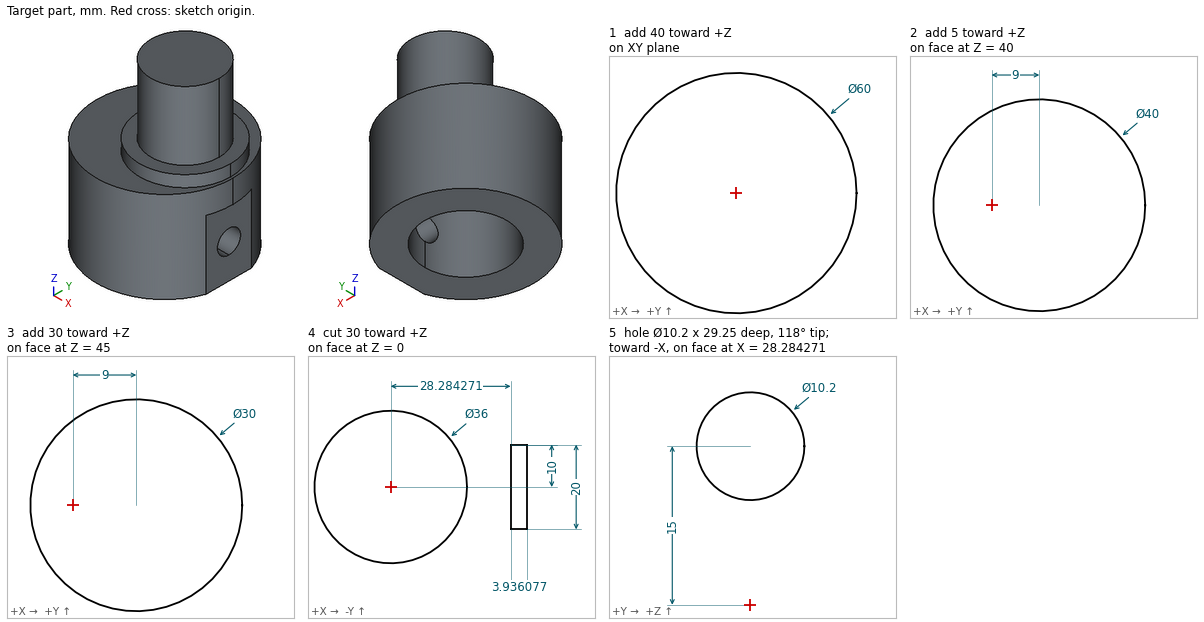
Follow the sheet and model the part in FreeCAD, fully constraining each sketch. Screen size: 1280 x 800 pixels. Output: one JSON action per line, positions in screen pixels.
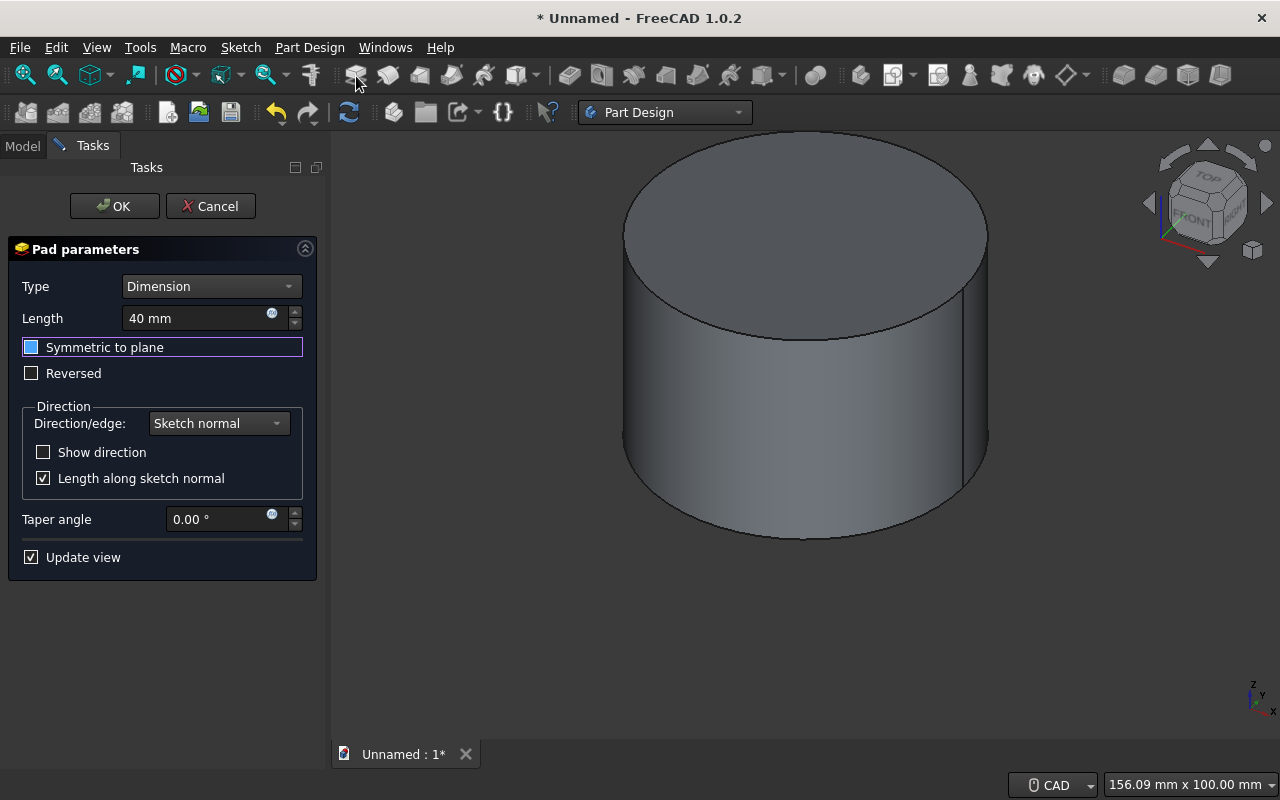
{"action": "left_click", "coordinate": [115, 206]}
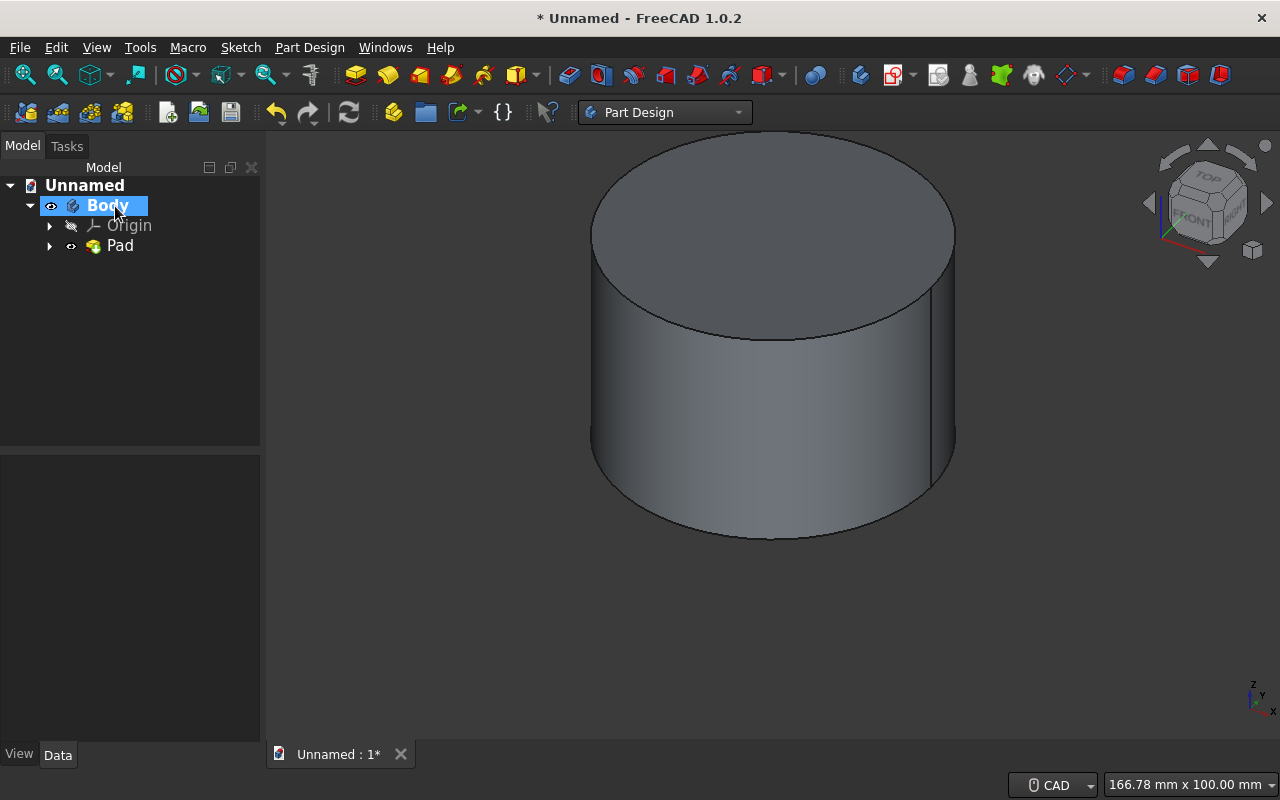
{"action": "key", "text": "v f"}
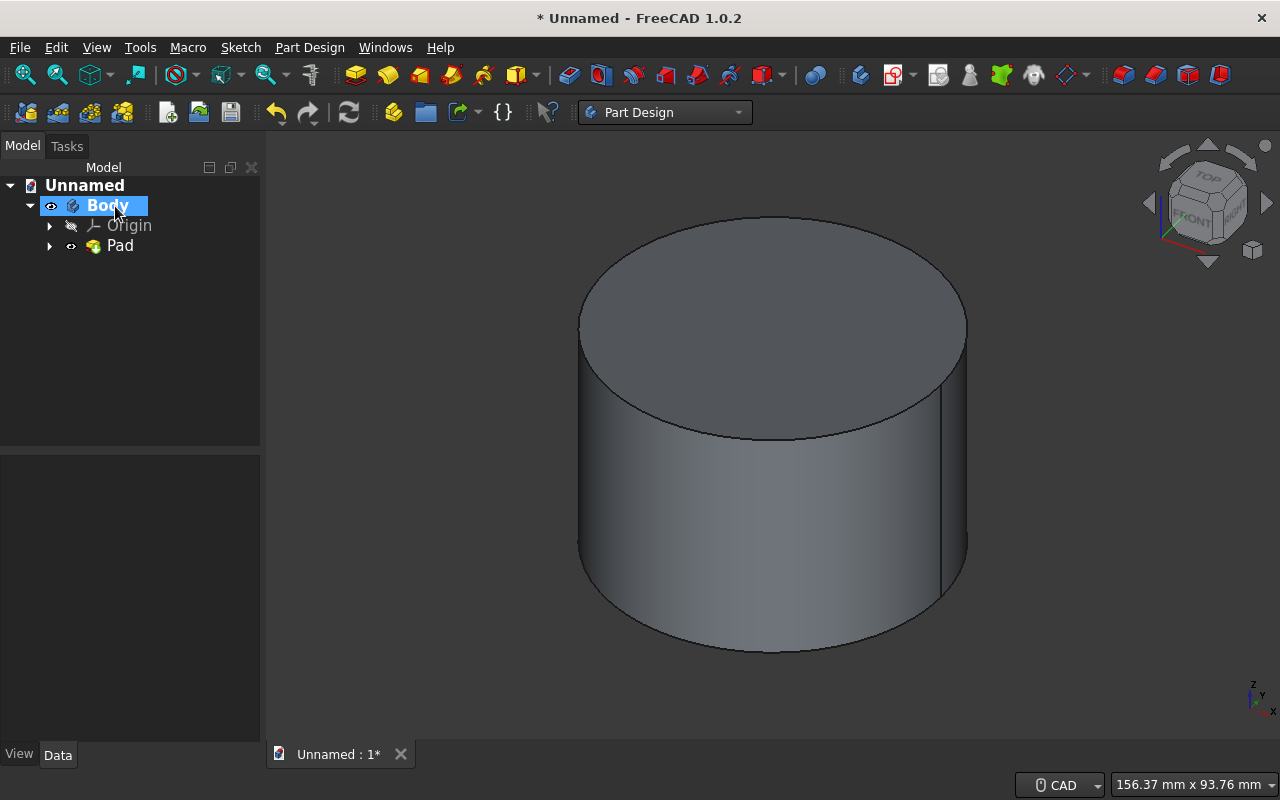
{"action": "left_click", "coordinate": [773, 328]}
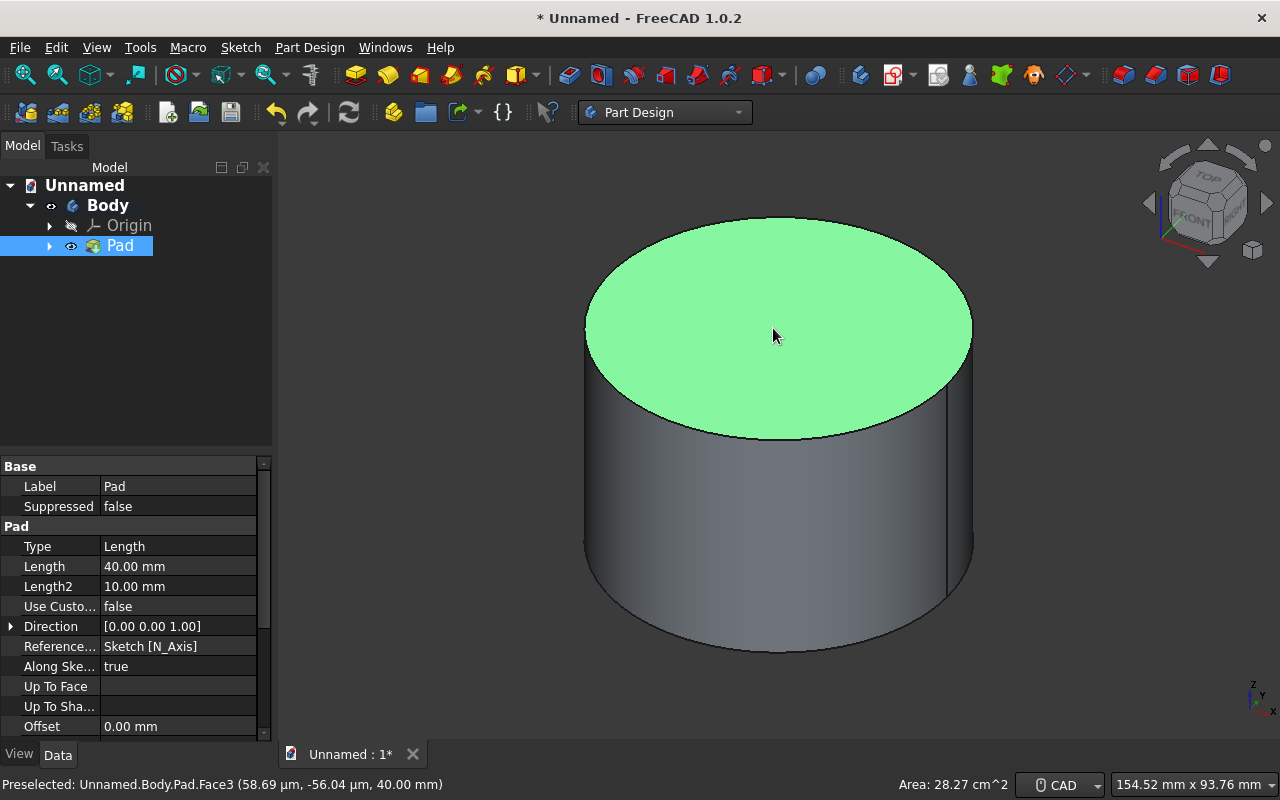
{"action": "left_click", "coordinate": [894, 76]}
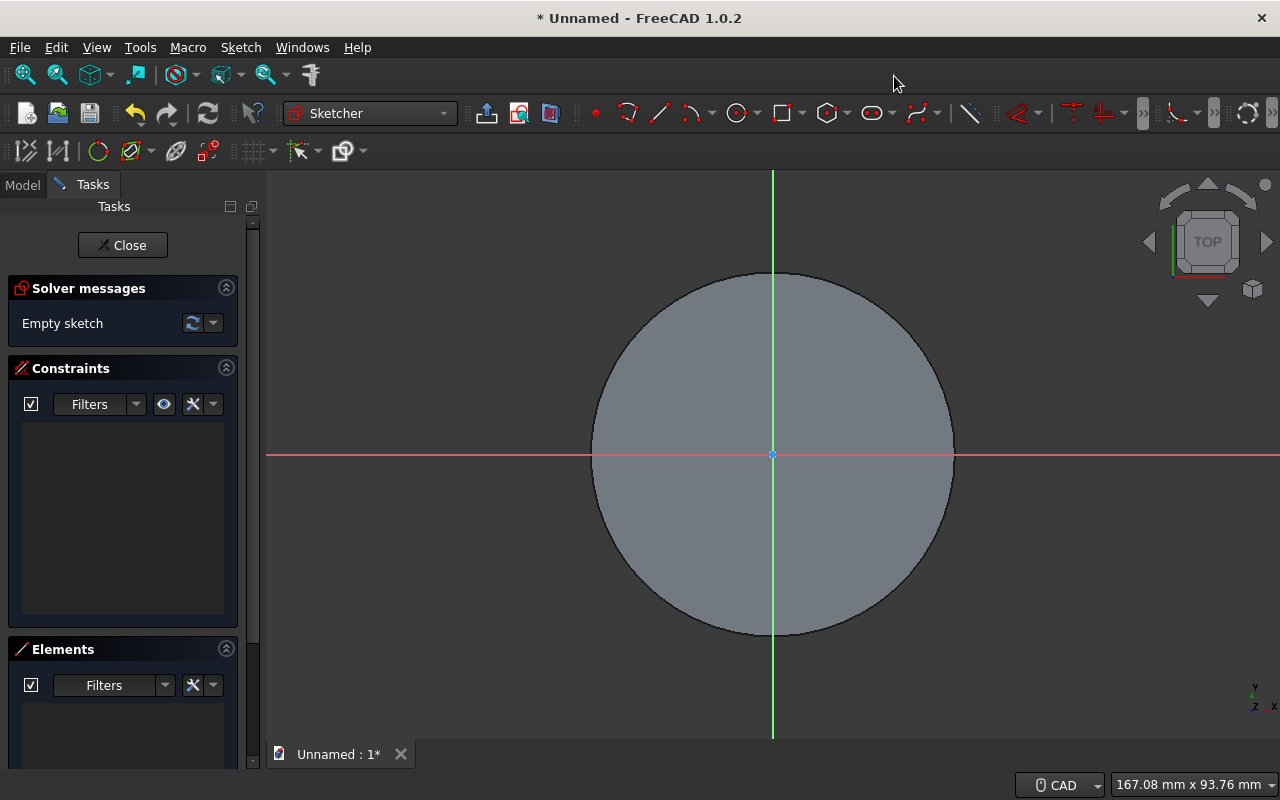
{"action": "scroll", "coordinate": [1077, 455], "scroll_direction": "up", "scroll_amount": 2}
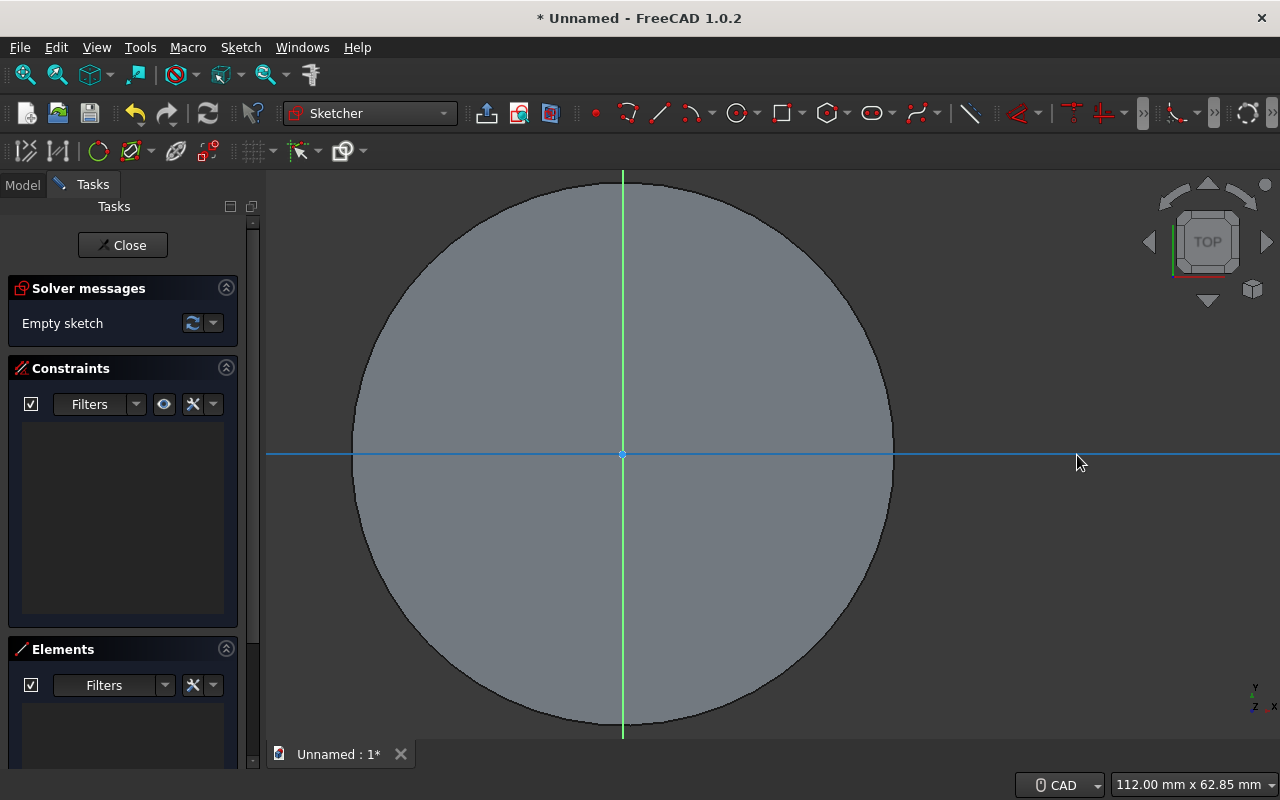
{"action": "left_click", "coordinate": [738, 114]}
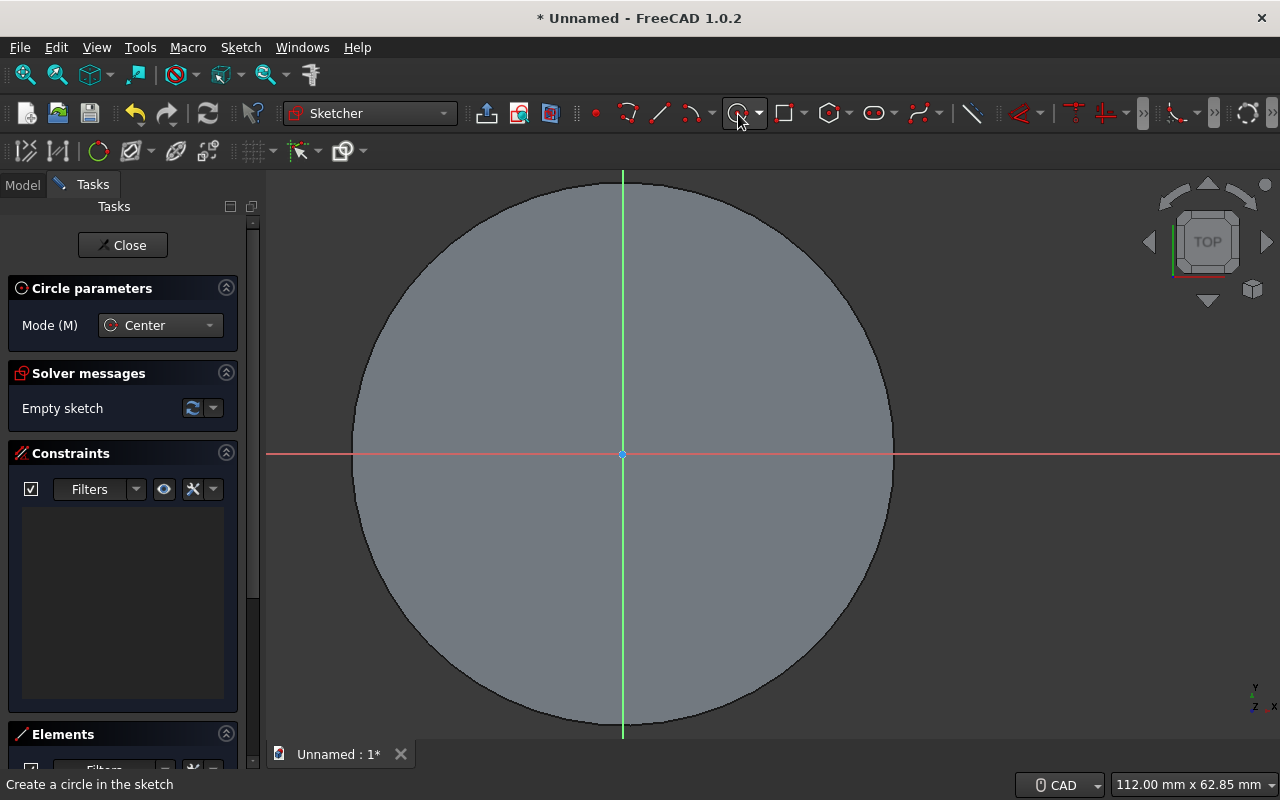
{"action": "left_click", "coordinate": [704, 454]}
{"action": "mouse_move", "coordinate": [832, 326]}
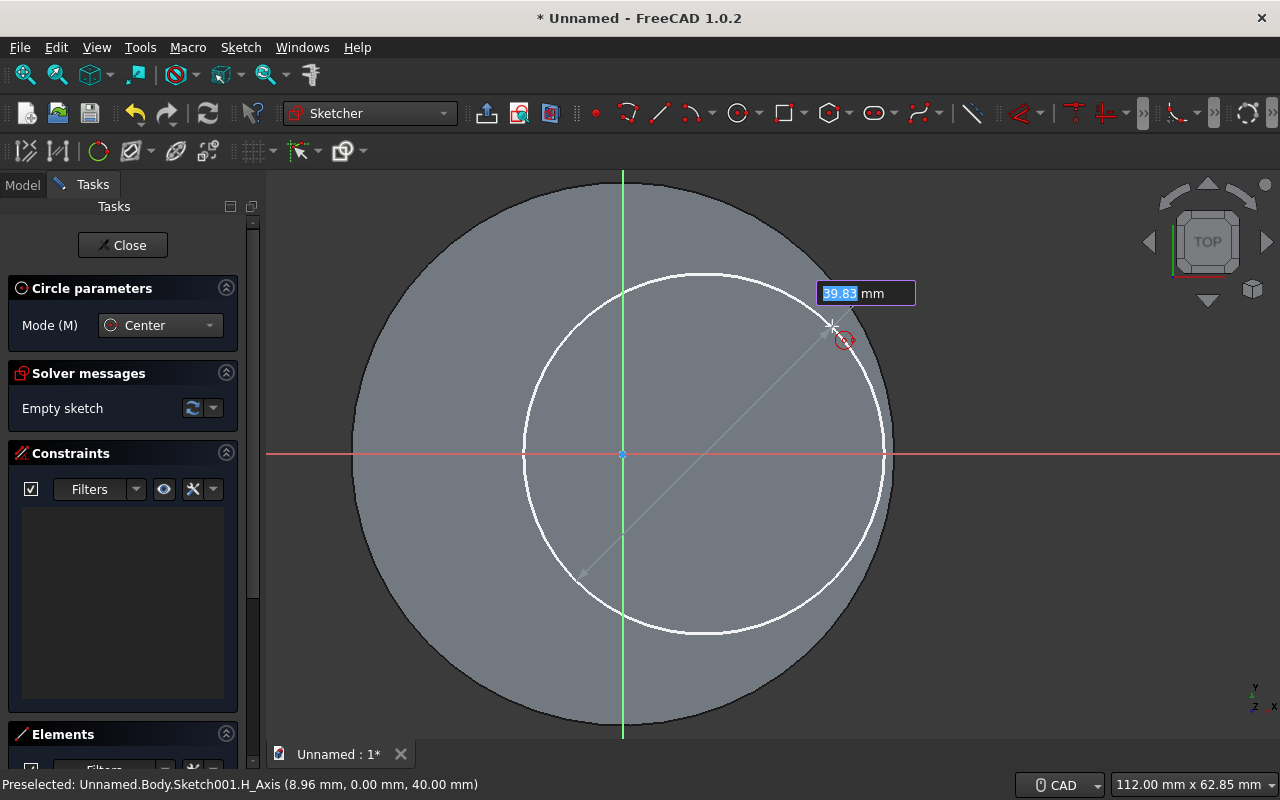
{"action": "type", "text": "40"}
{"action": "key", "text": "Return"}
{"action": "key", "text": "Escape"}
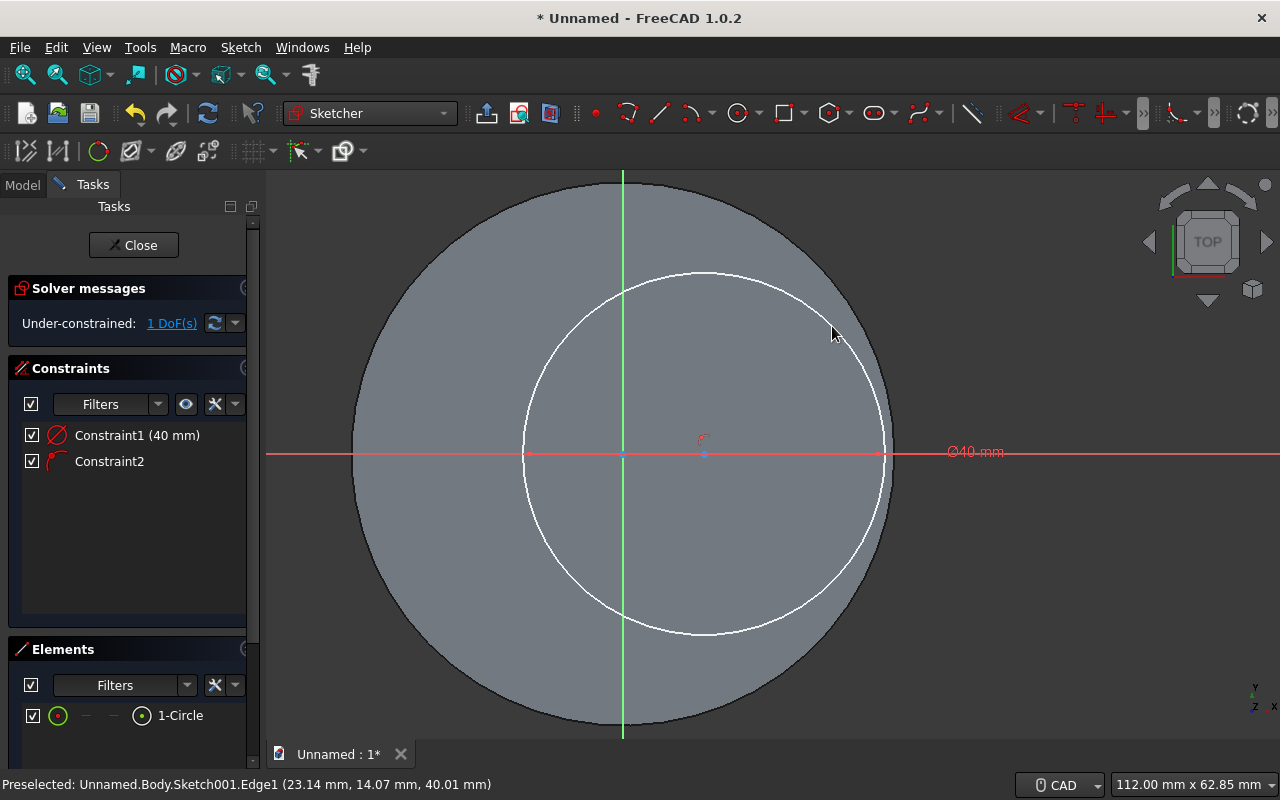
{"action": "key", "text": "d"}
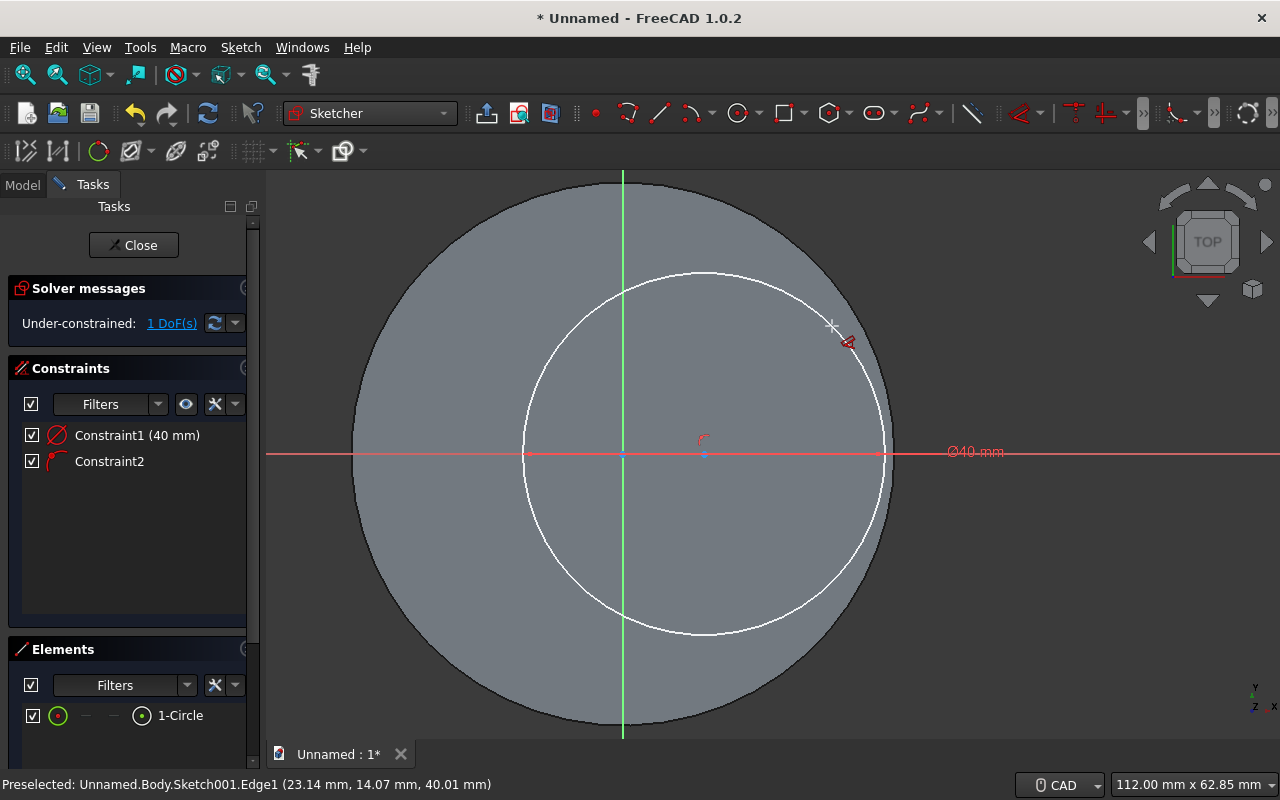
{"action": "left_click", "coordinate": [704, 454]}
{"action": "left_click", "coordinate": [663, 488]}